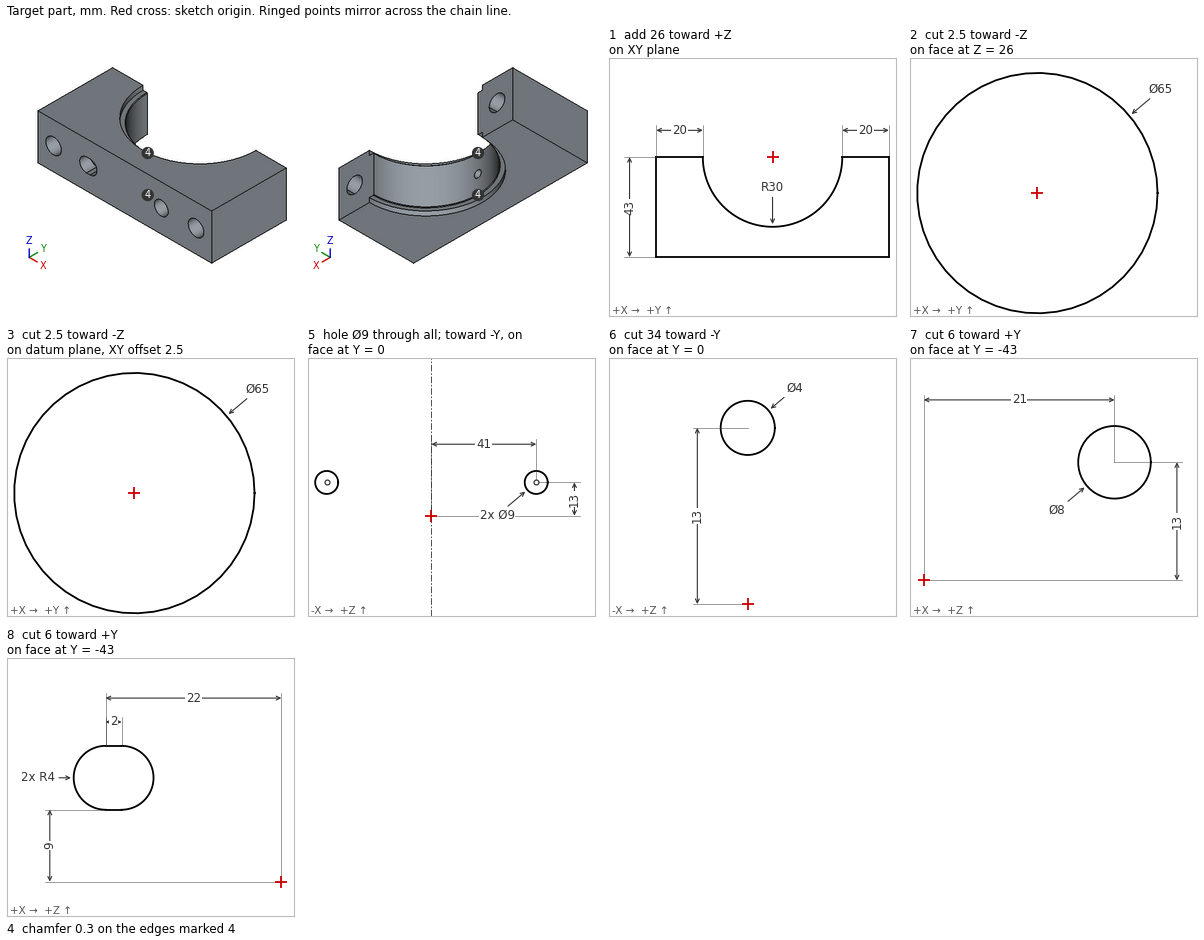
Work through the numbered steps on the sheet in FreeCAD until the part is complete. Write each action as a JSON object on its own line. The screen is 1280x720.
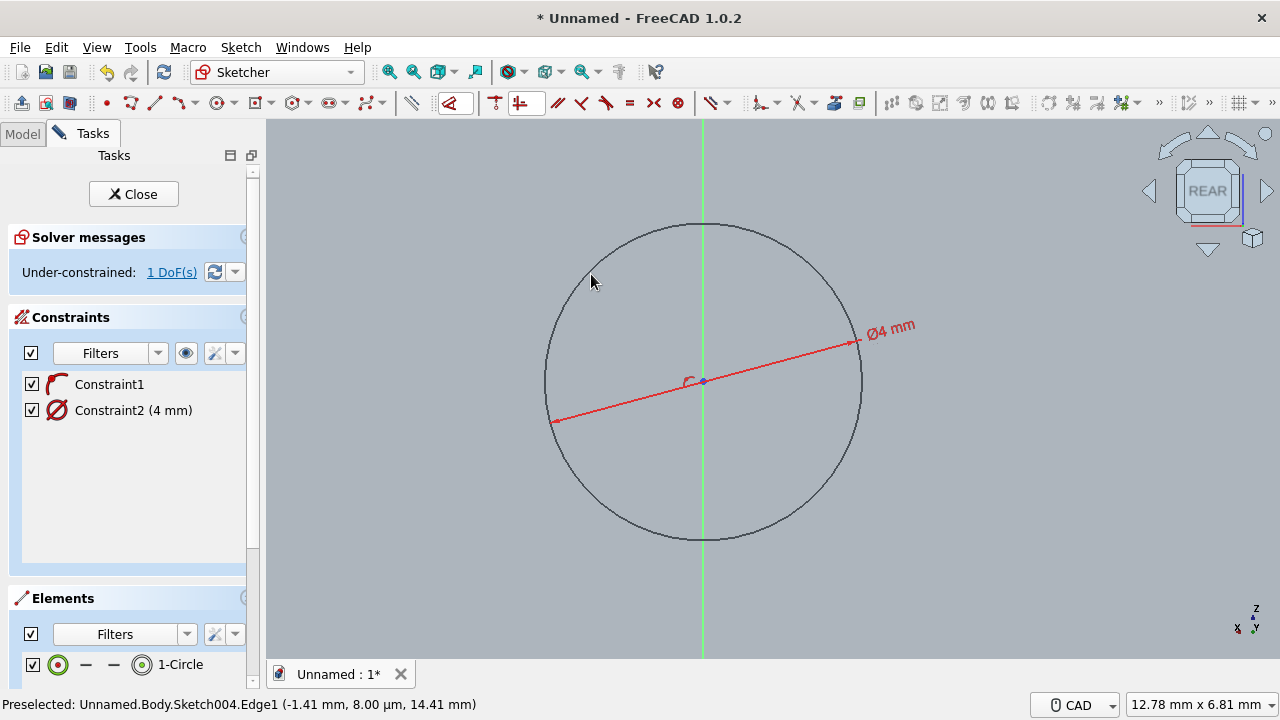
{"action": "left_click", "coordinate": [703, 382]}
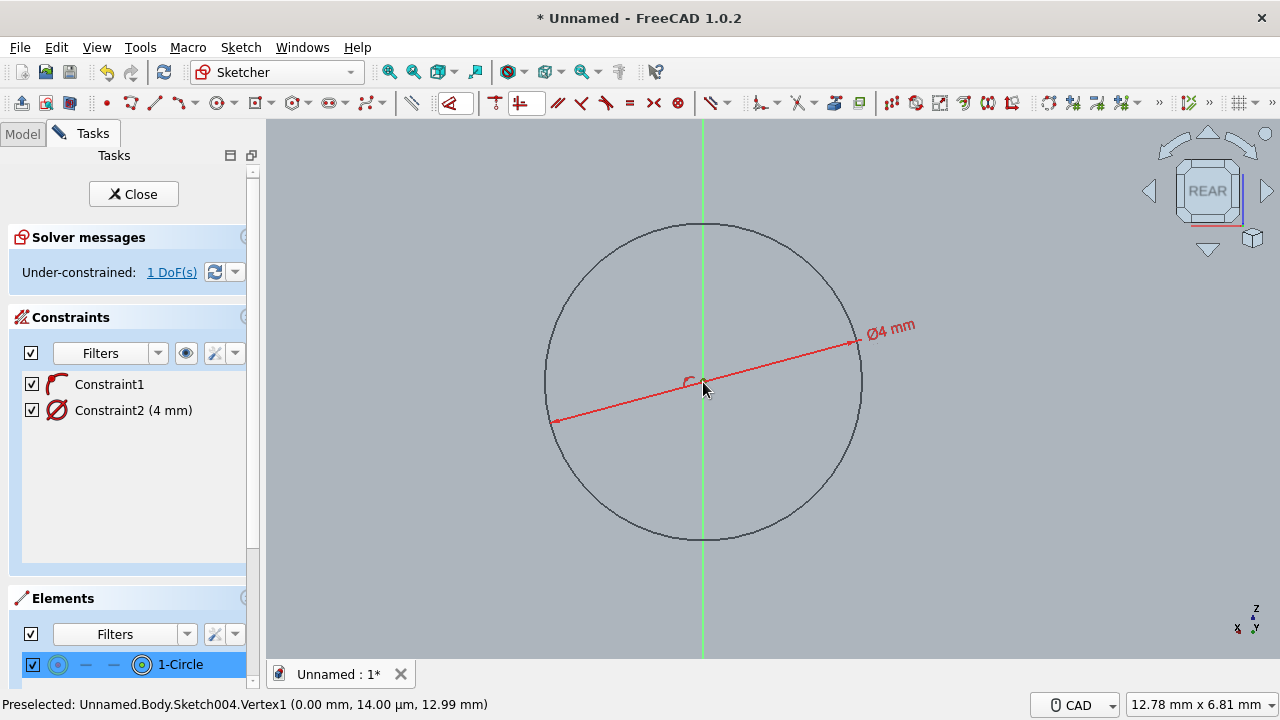
{"action": "left_click", "coordinate": [468, 104]}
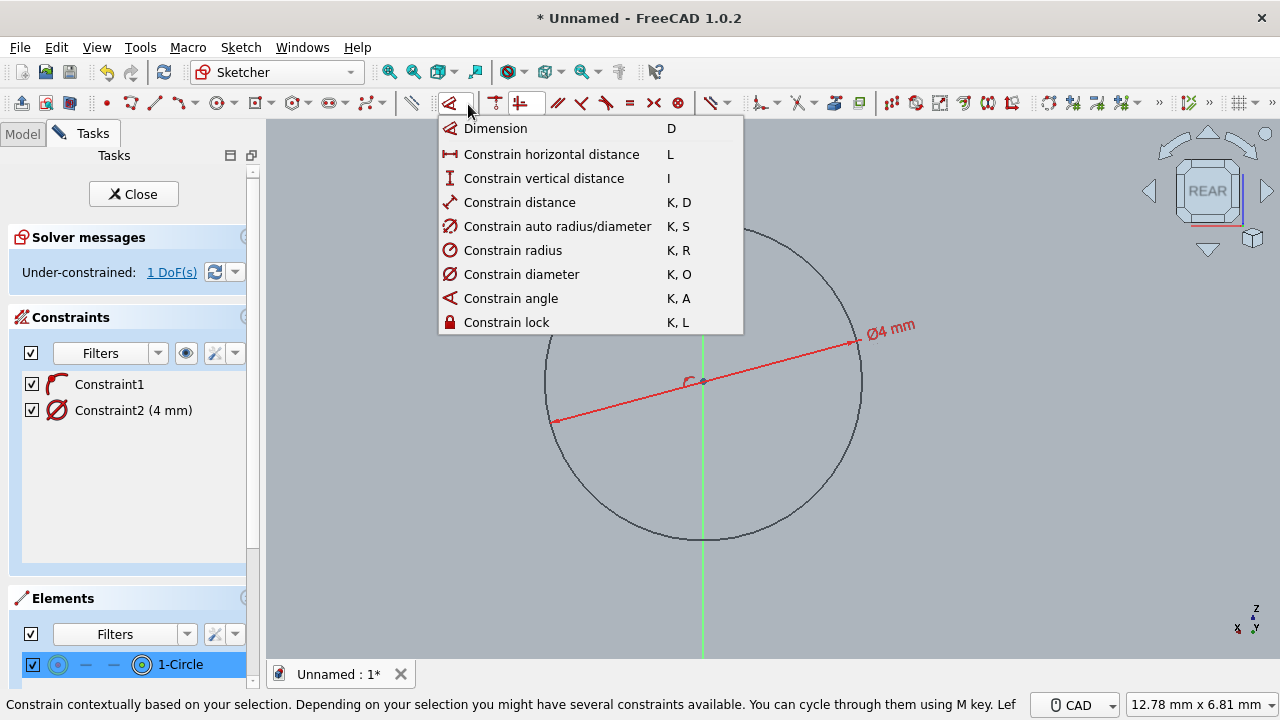
{"action": "left_click", "coordinate": [591, 178]}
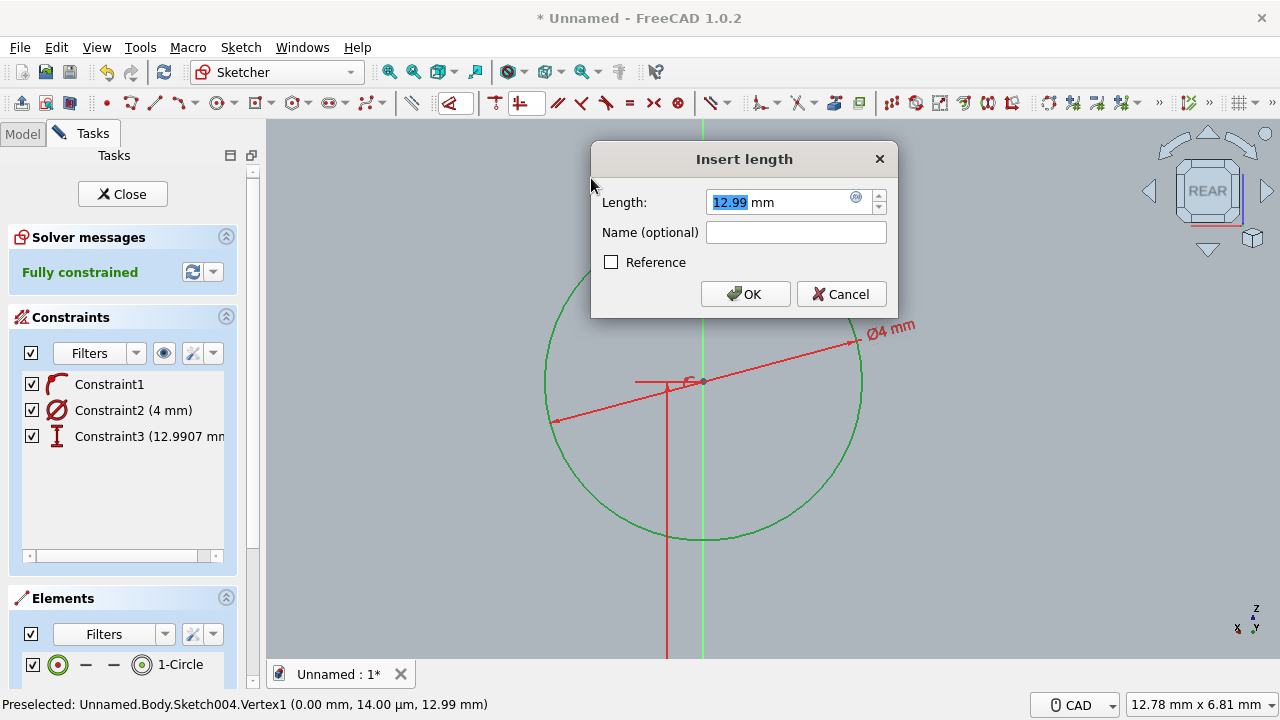
{"action": "type", "text": "13"}
{"action": "key", "text": "Return"}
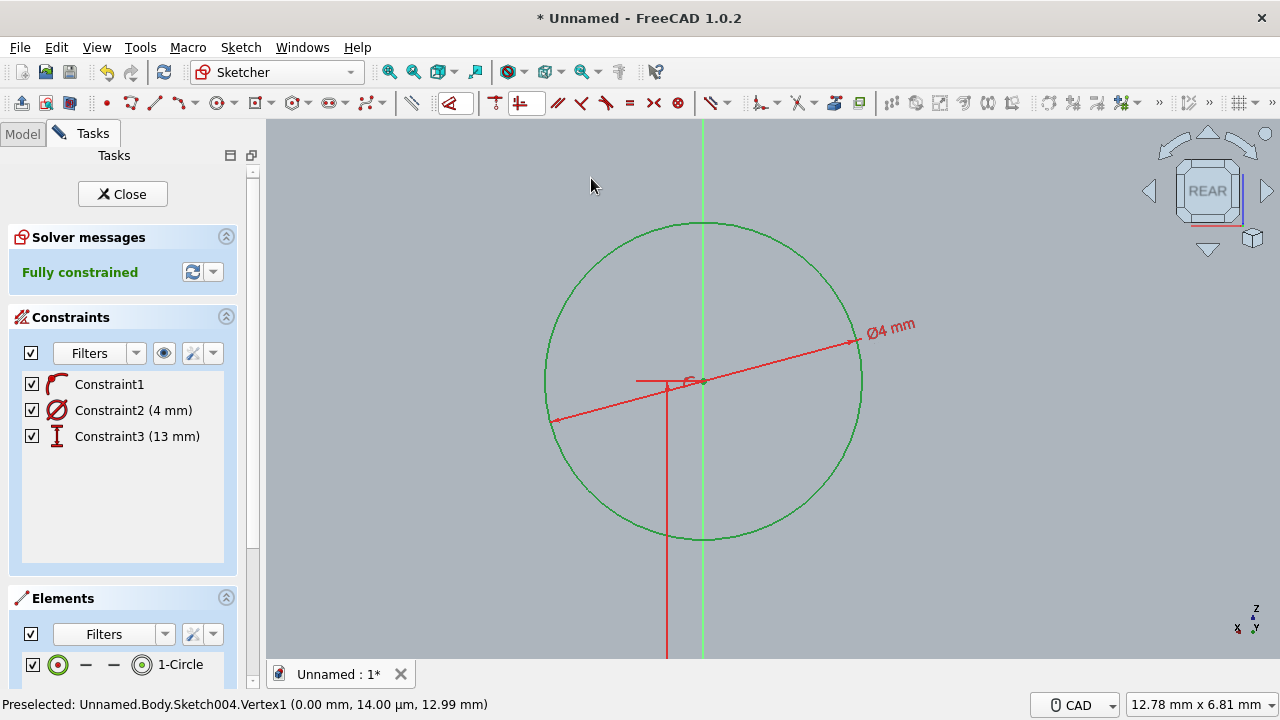
{"action": "left_click", "coordinate": [123, 194]}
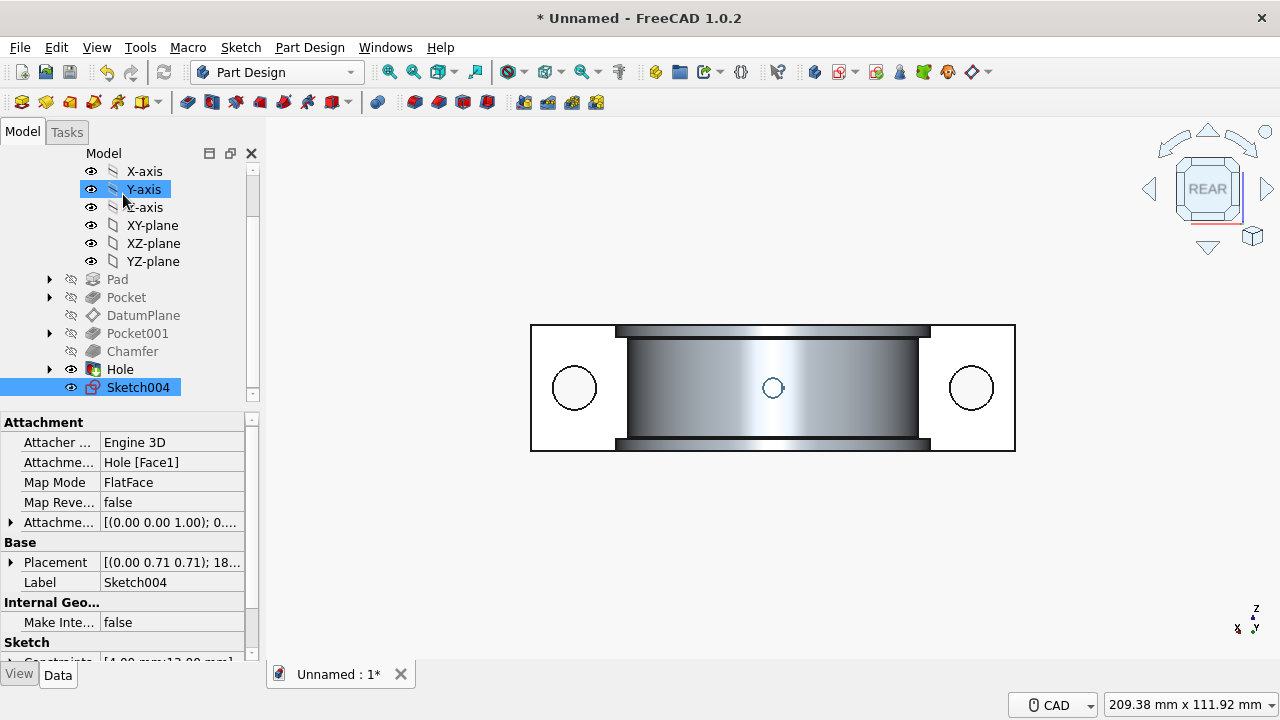
{"action": "left_click", "coordinate": [188, 102]}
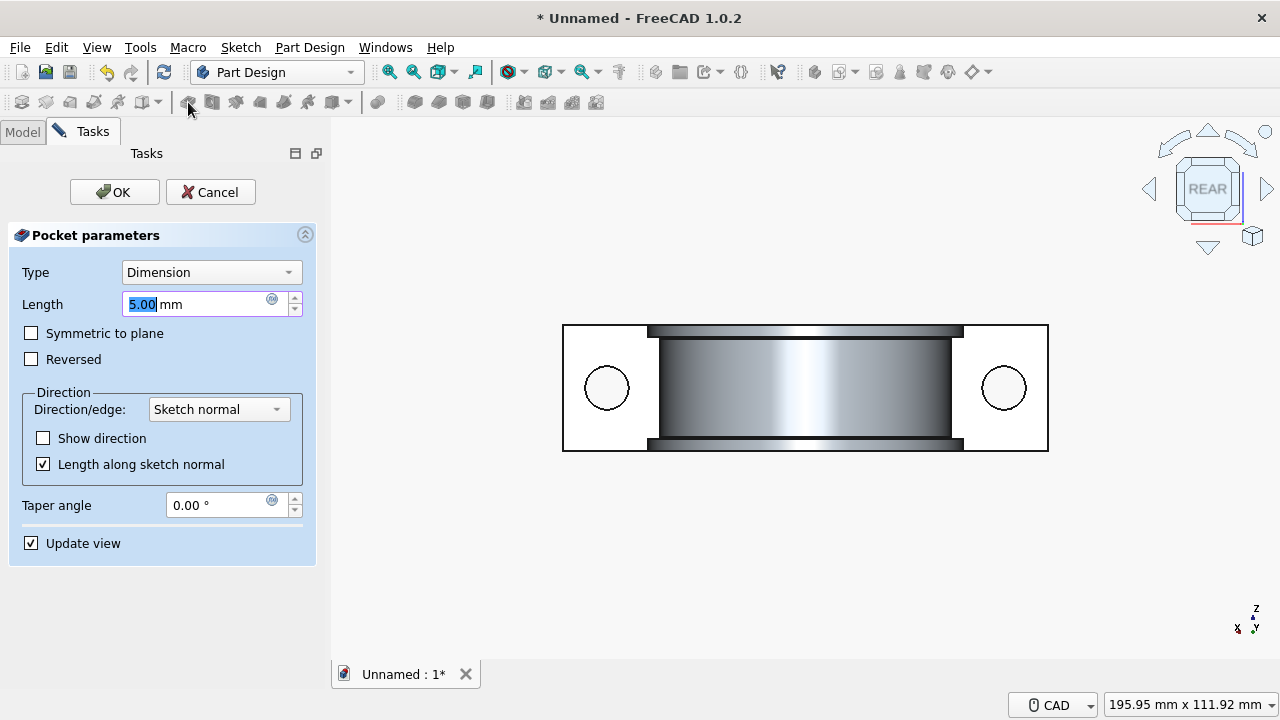
{"action": "type", "text": "34"}
{"action": "key", "text": "Tab"}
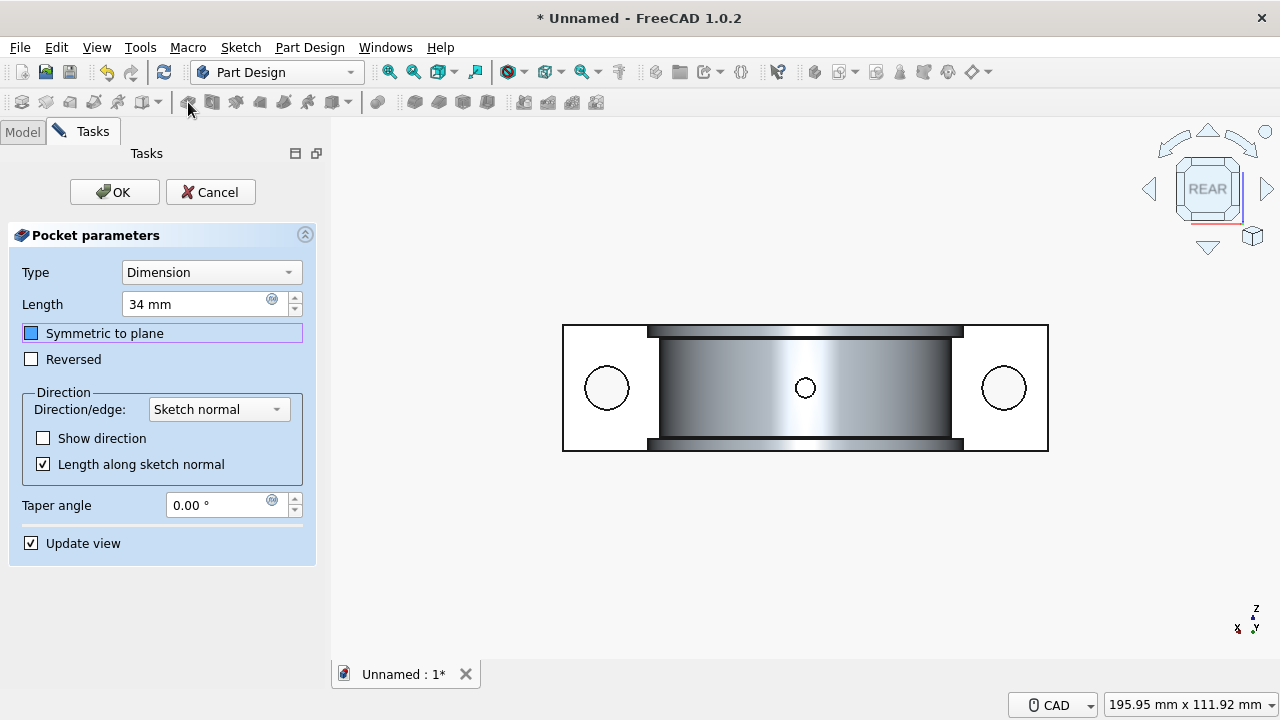
{"action": "left_click", "coordinate": [115, 192]}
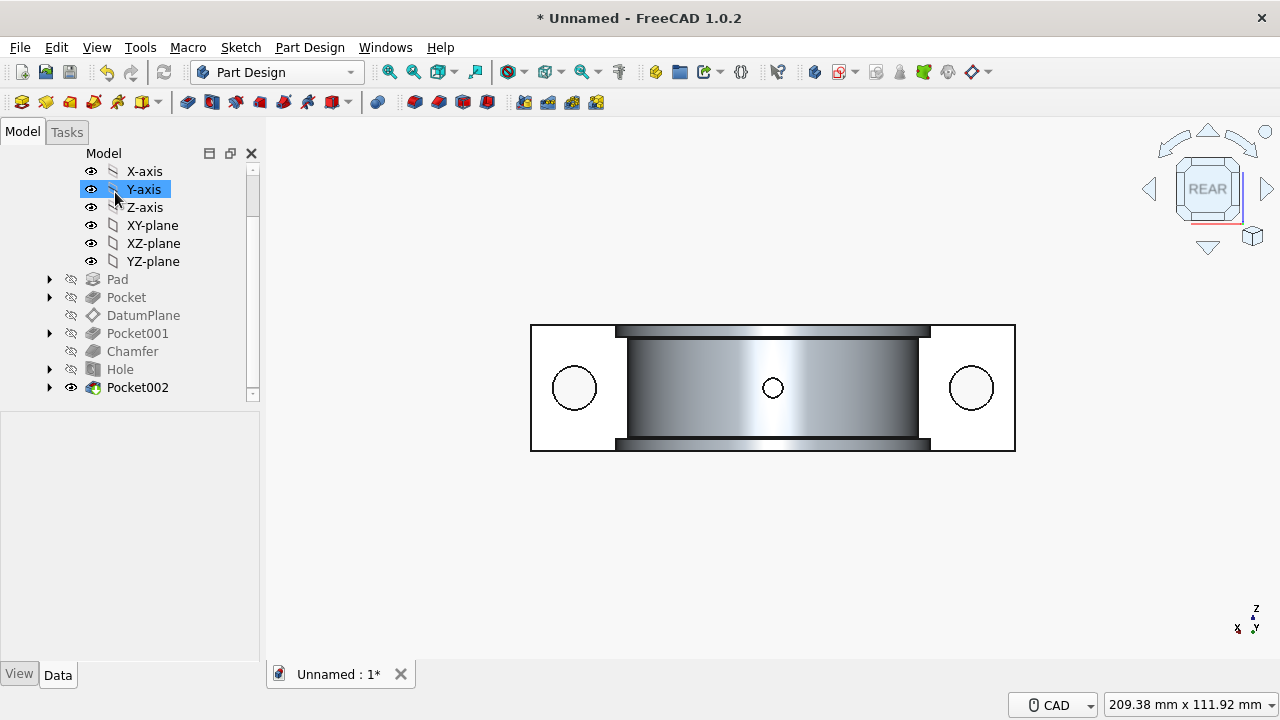
{"action": "key", "text": "0"}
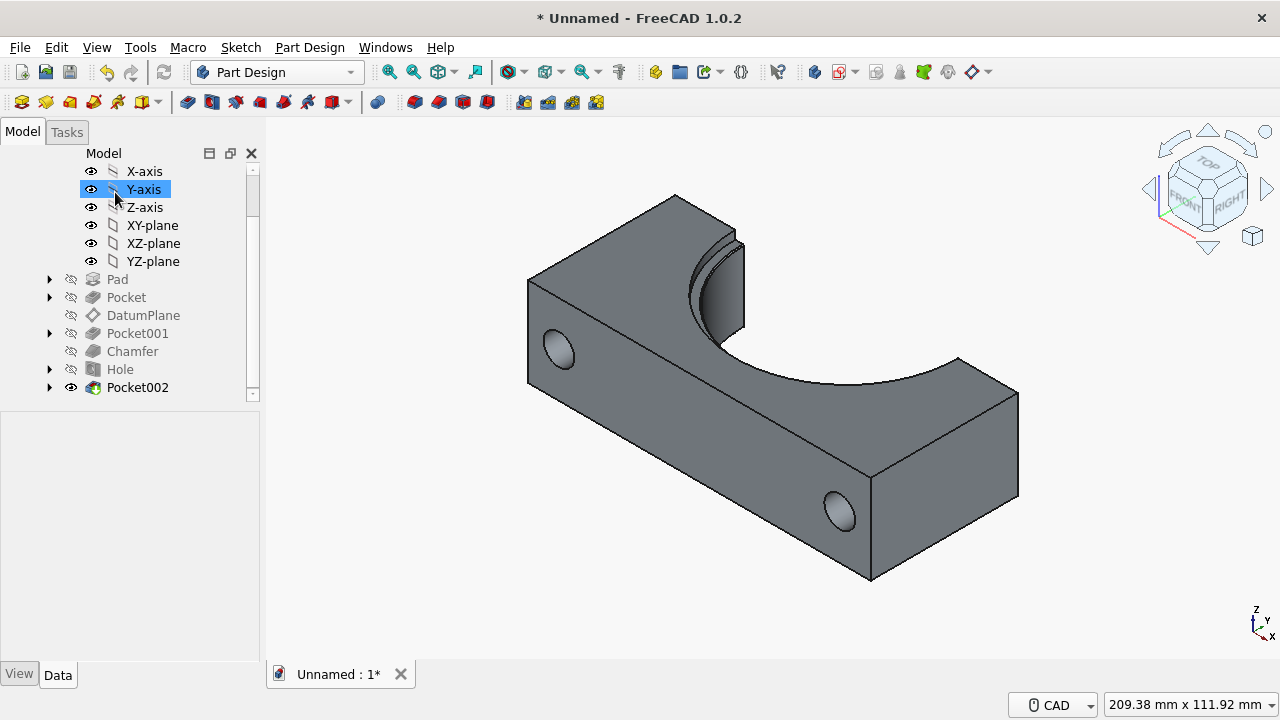
{"action": "left_click", "coordinate": [748, 458]}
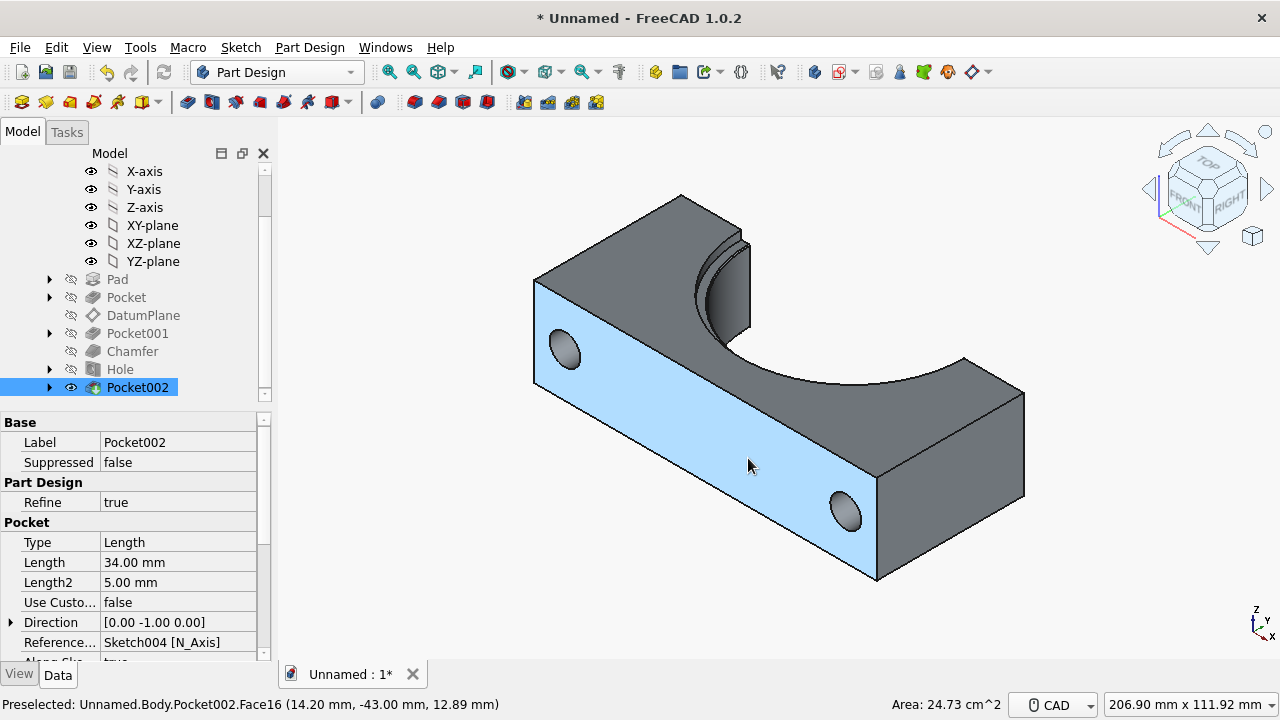
{"action": "left_click", "coordinate": [840, 72]}